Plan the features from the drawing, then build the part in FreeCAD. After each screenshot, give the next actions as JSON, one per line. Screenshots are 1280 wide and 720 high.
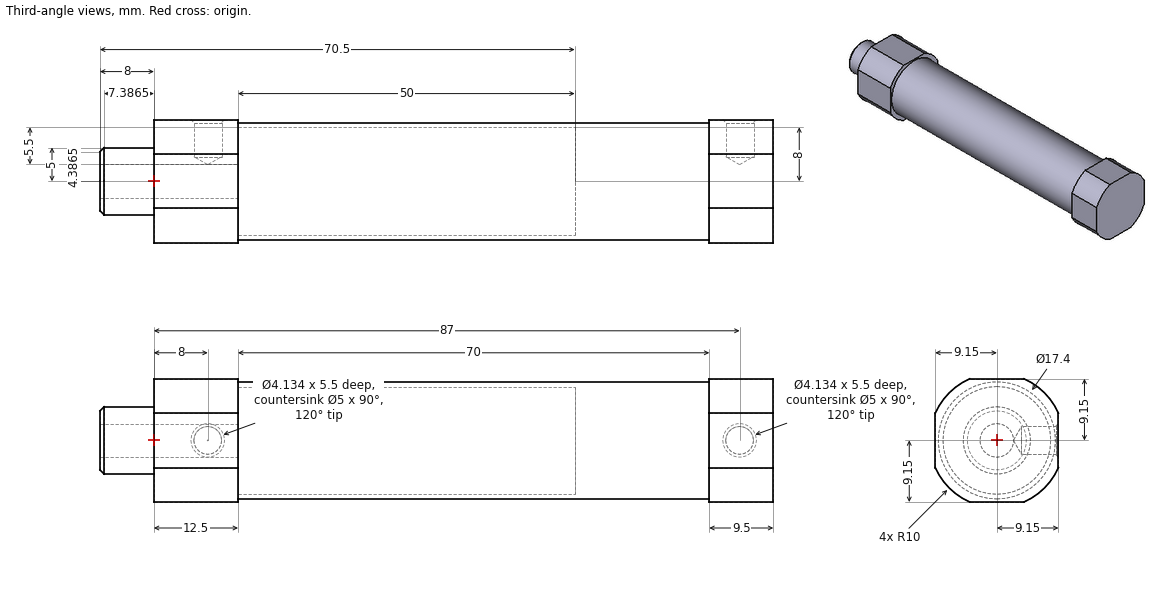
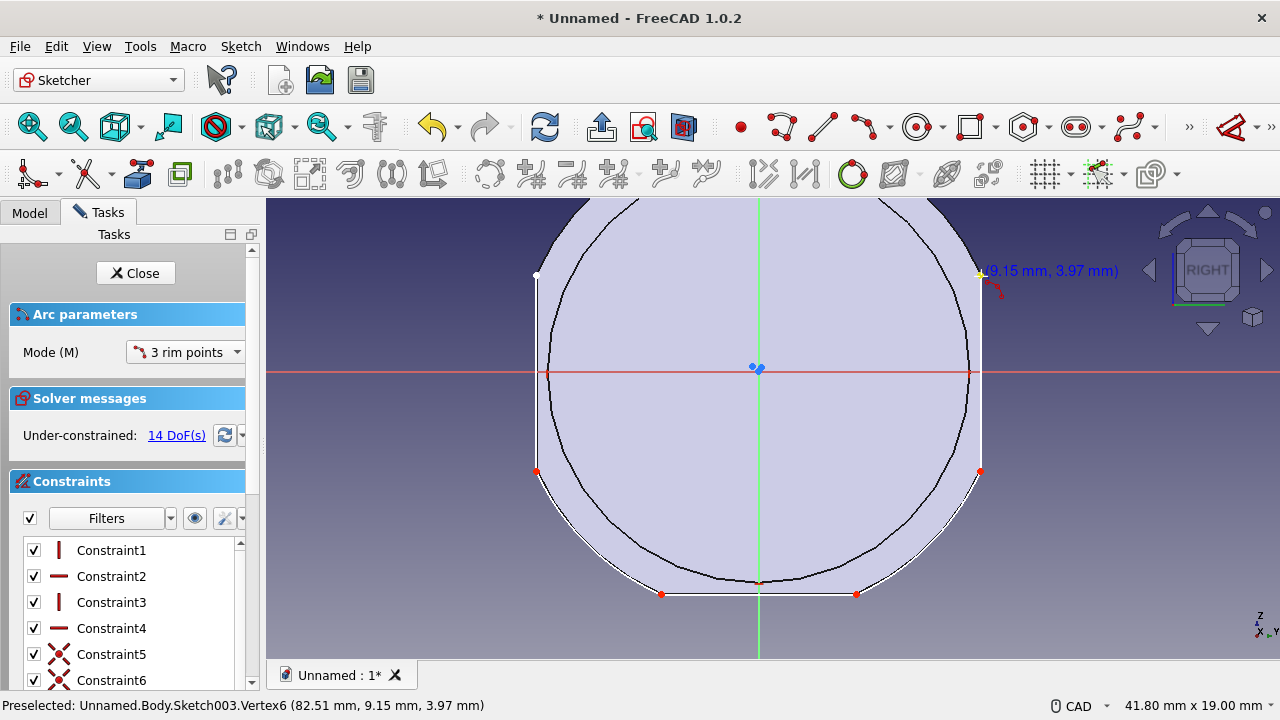
{"action": "scroll", "coordinate": [594, 544], "scroll_direction": "down", "scroll_amount": 2}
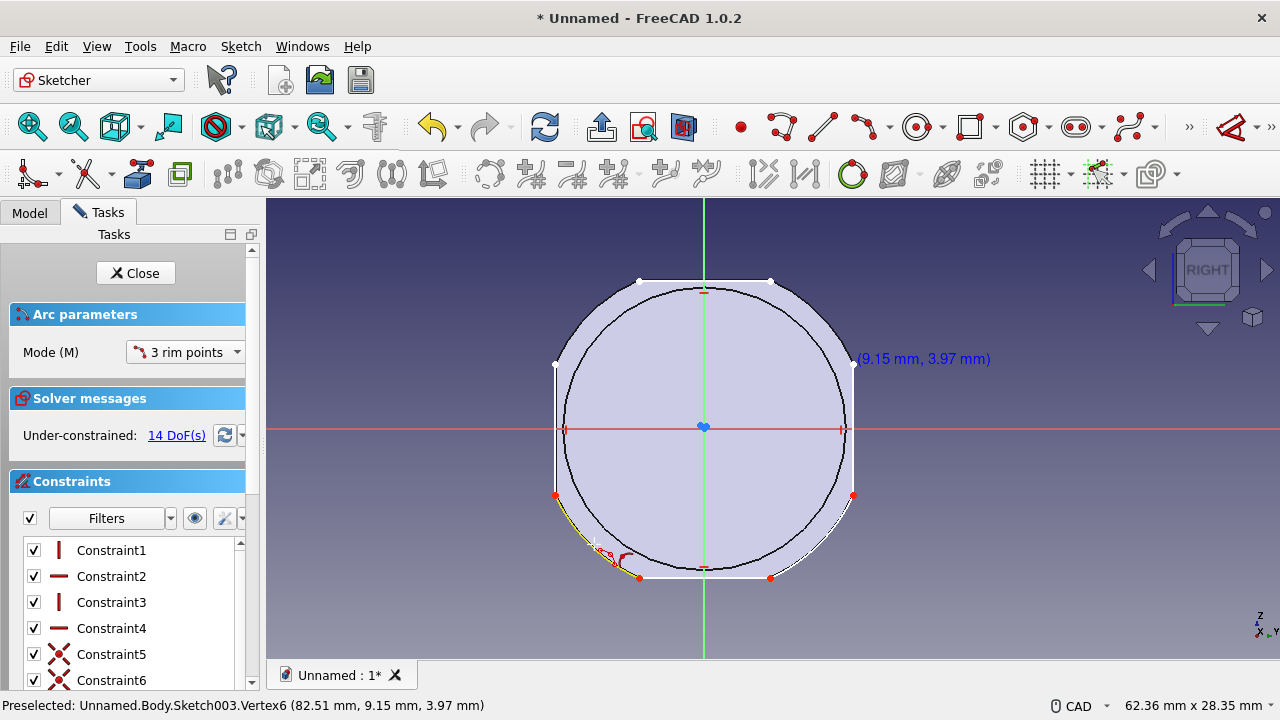
{"action": "left_click", "coordinate": [770, 281]}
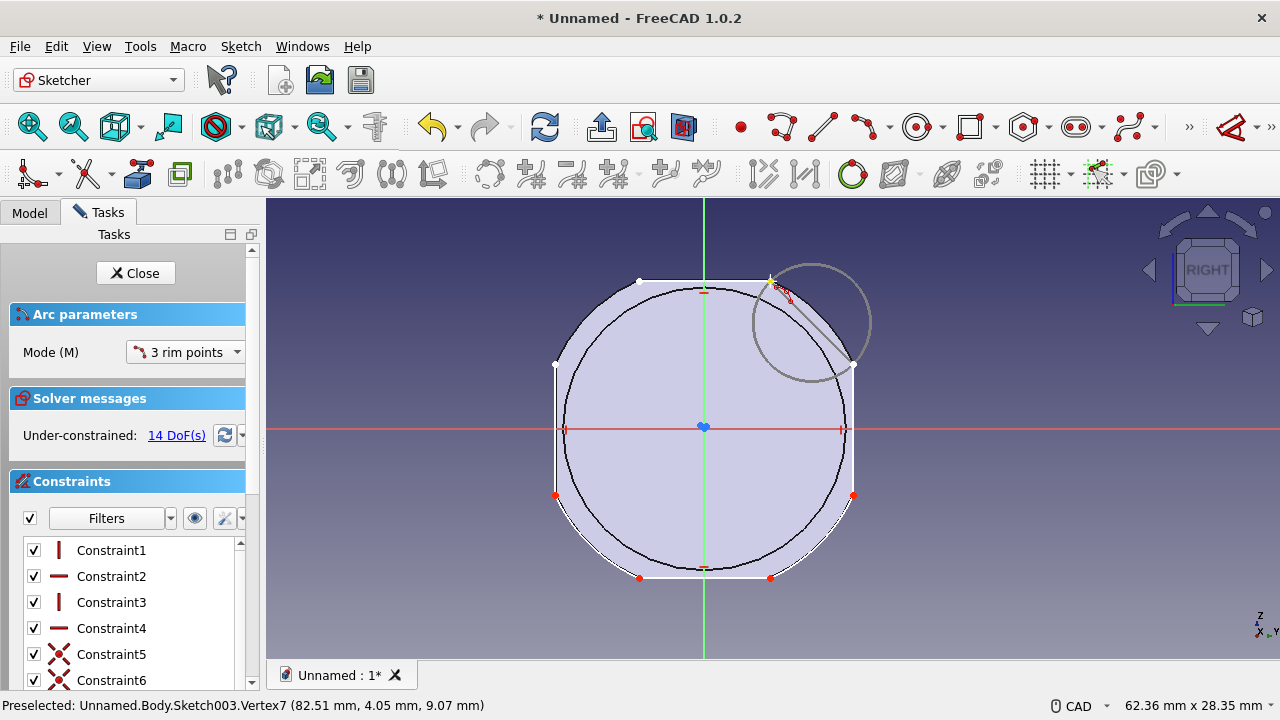
{"action": "scroll", "coordinate": [819, 314], "scroll_direction": "up", "scroll_amount": 2}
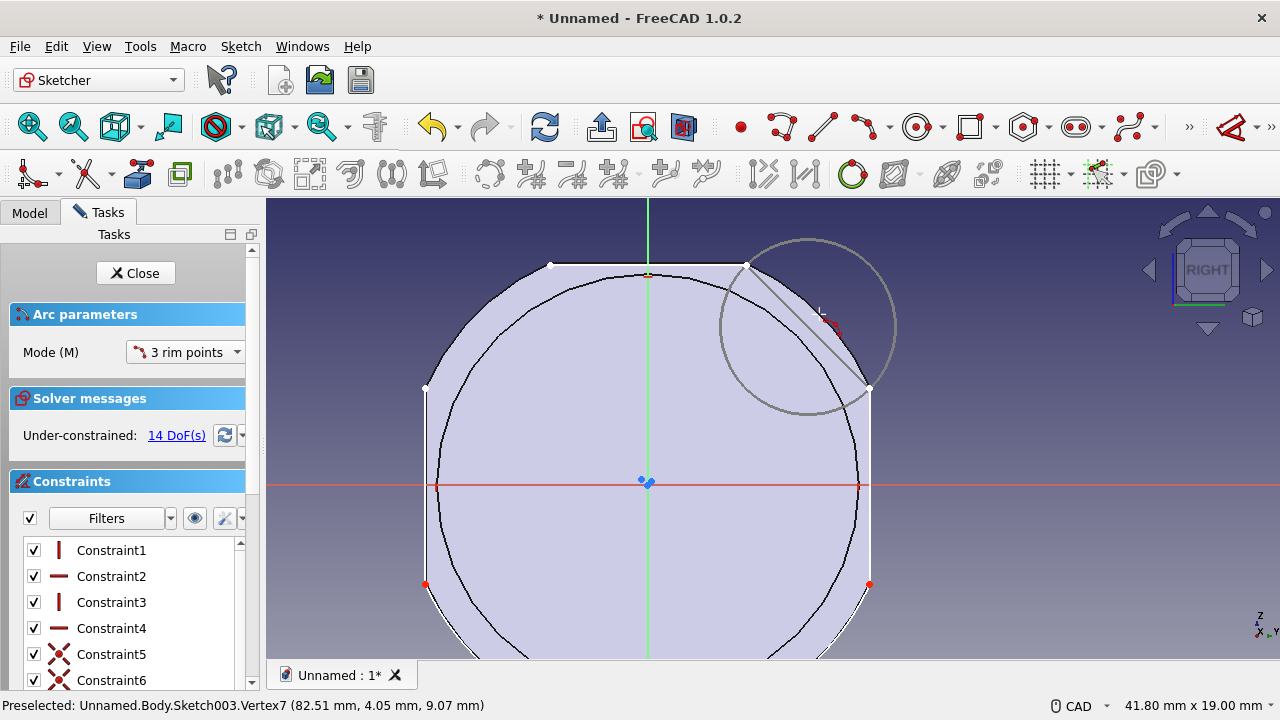
{"action": "left_click", "coordinate": [819, 314]}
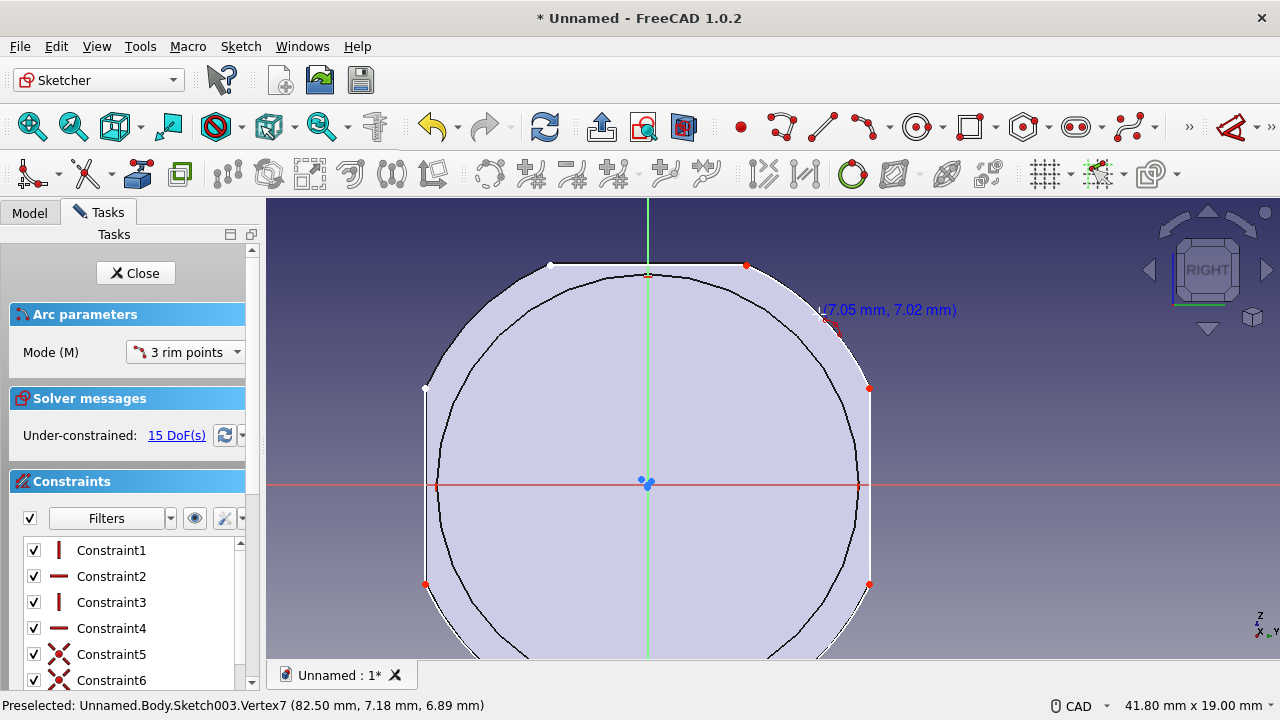
{"action": "left_click", "coordinate": [551, 265]}
{"action": "left_click", "coordinate": [425, 389]}
{"action": "left_click", "coordinate": [476, 314]}
{"action": "key", "text": "Escape"}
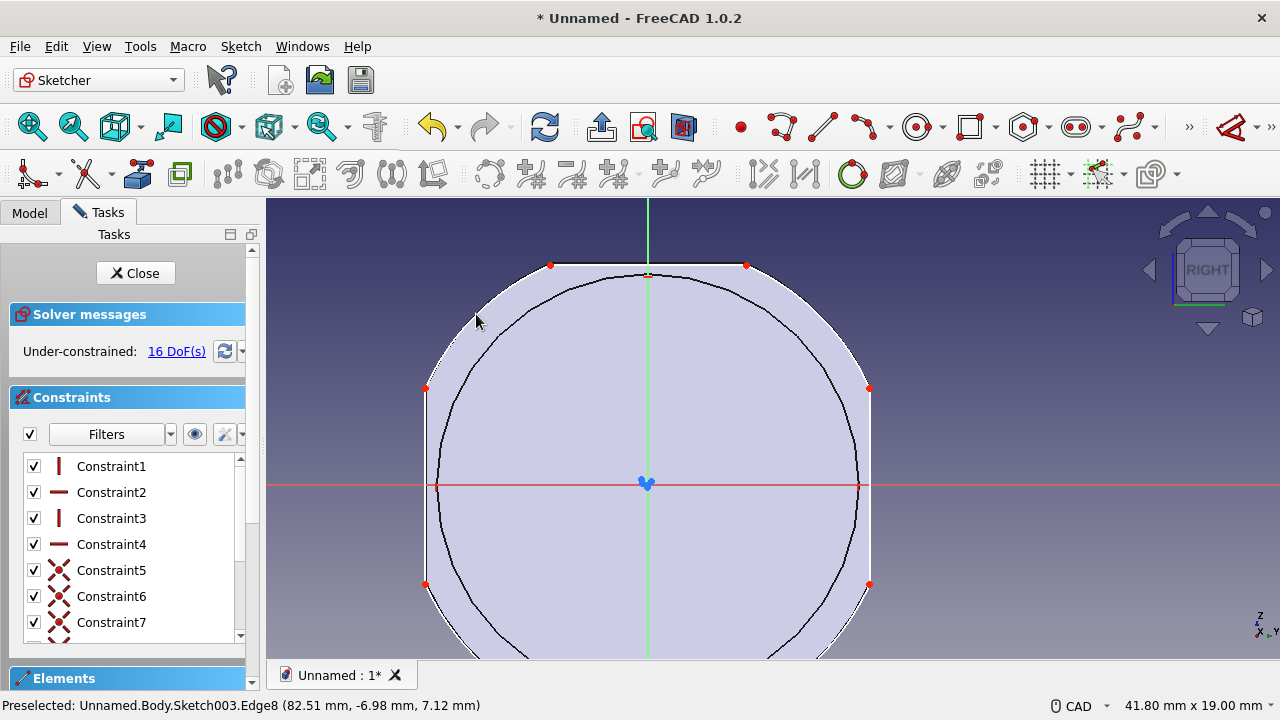
{"action": "left_click", "coordinate": [453, 631]}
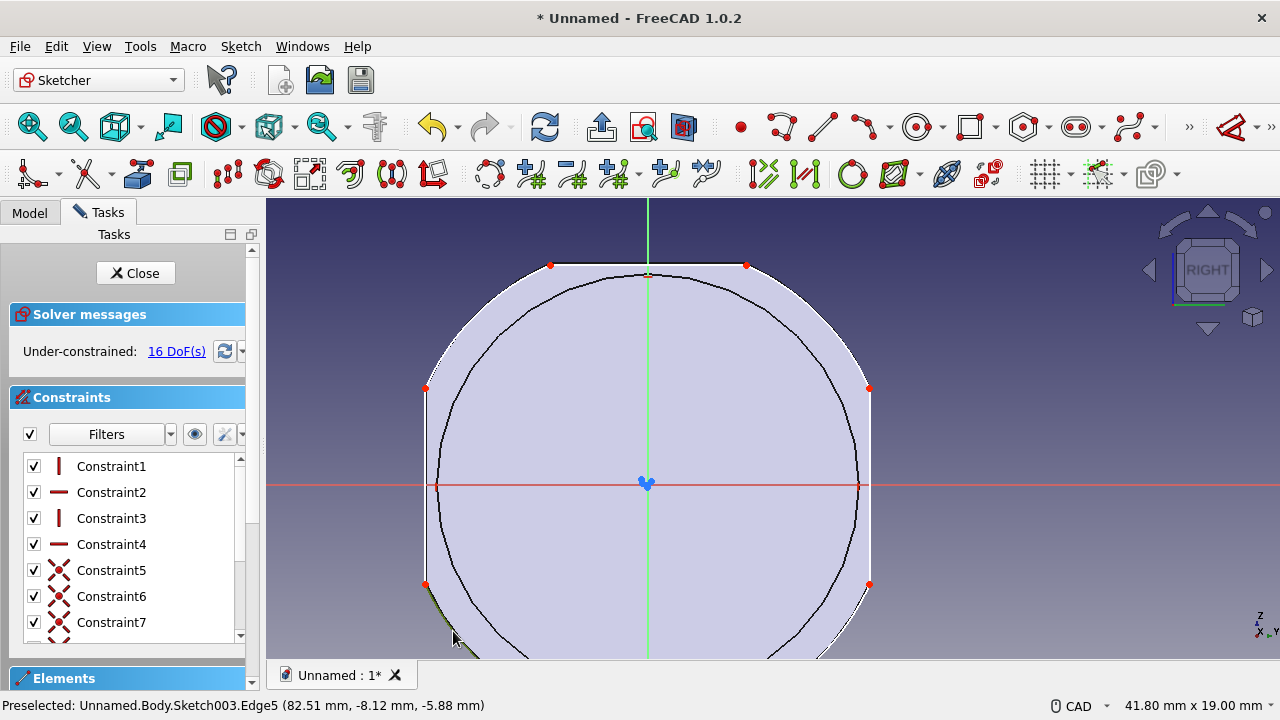
{"action": "left_click", "coordinate": [843, 630]}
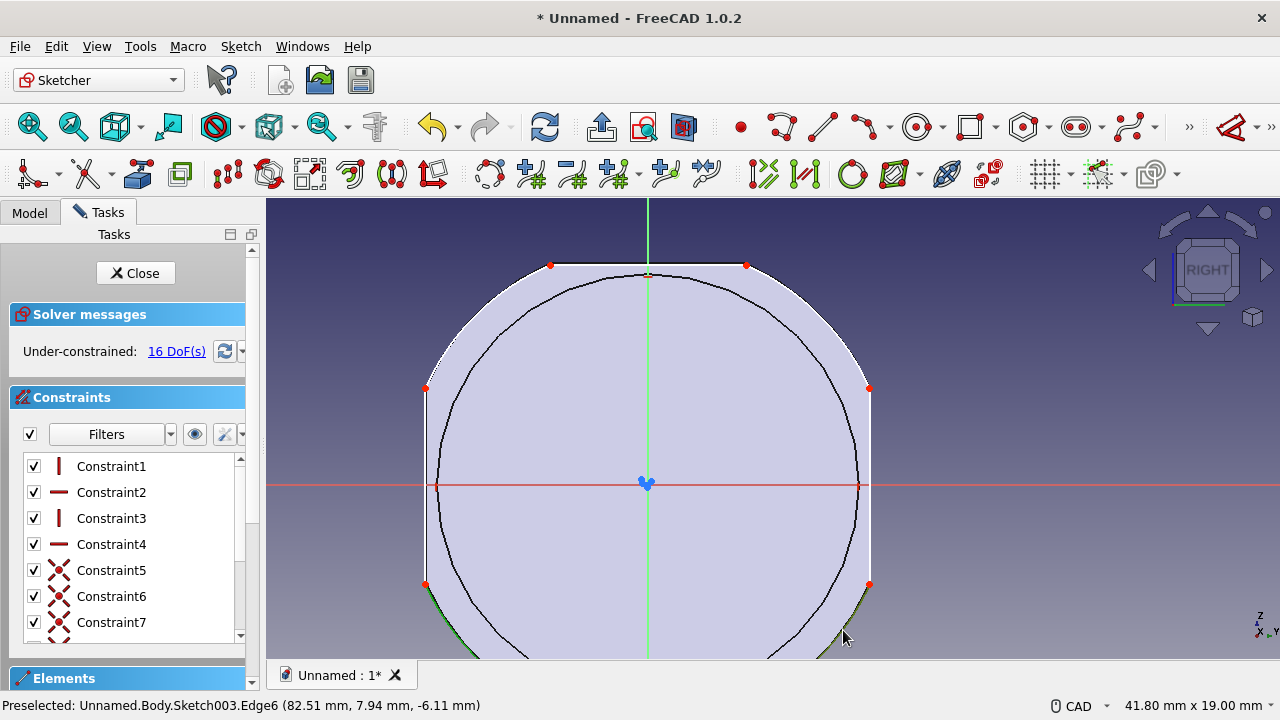
{"action": "key", "text": "c"}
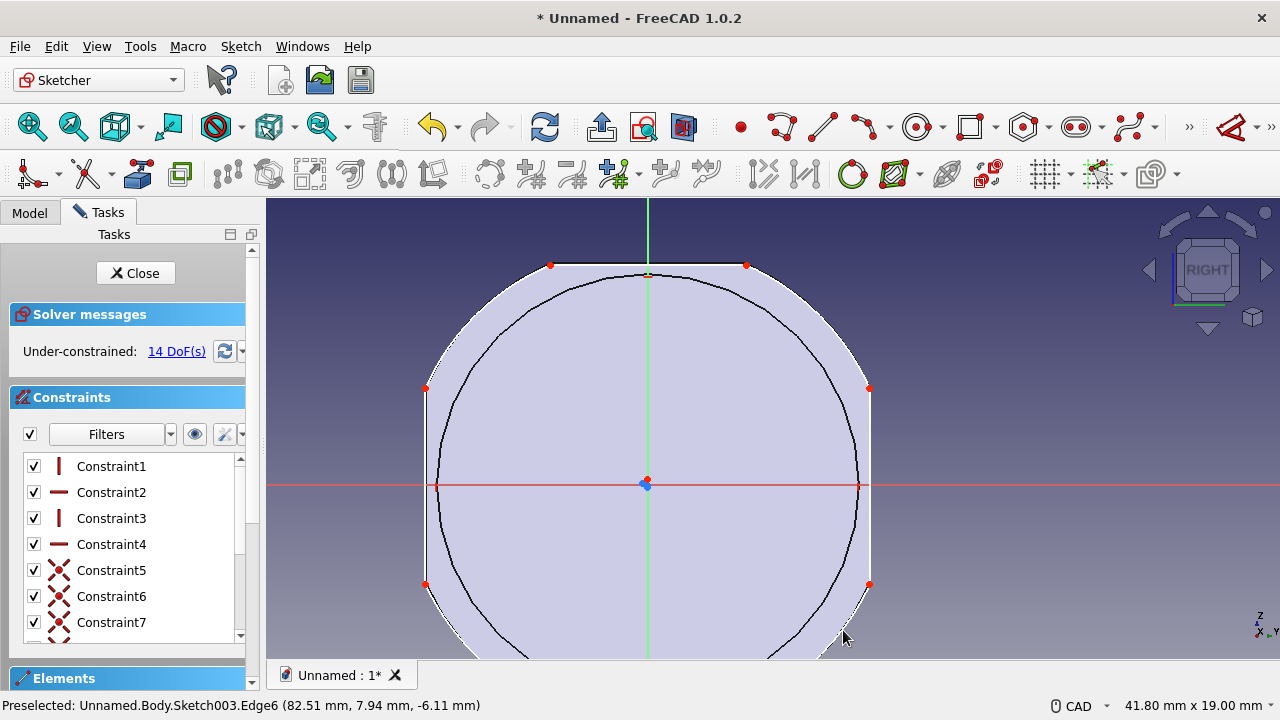
{"action": "left_click", "coordinate": [453, 630]}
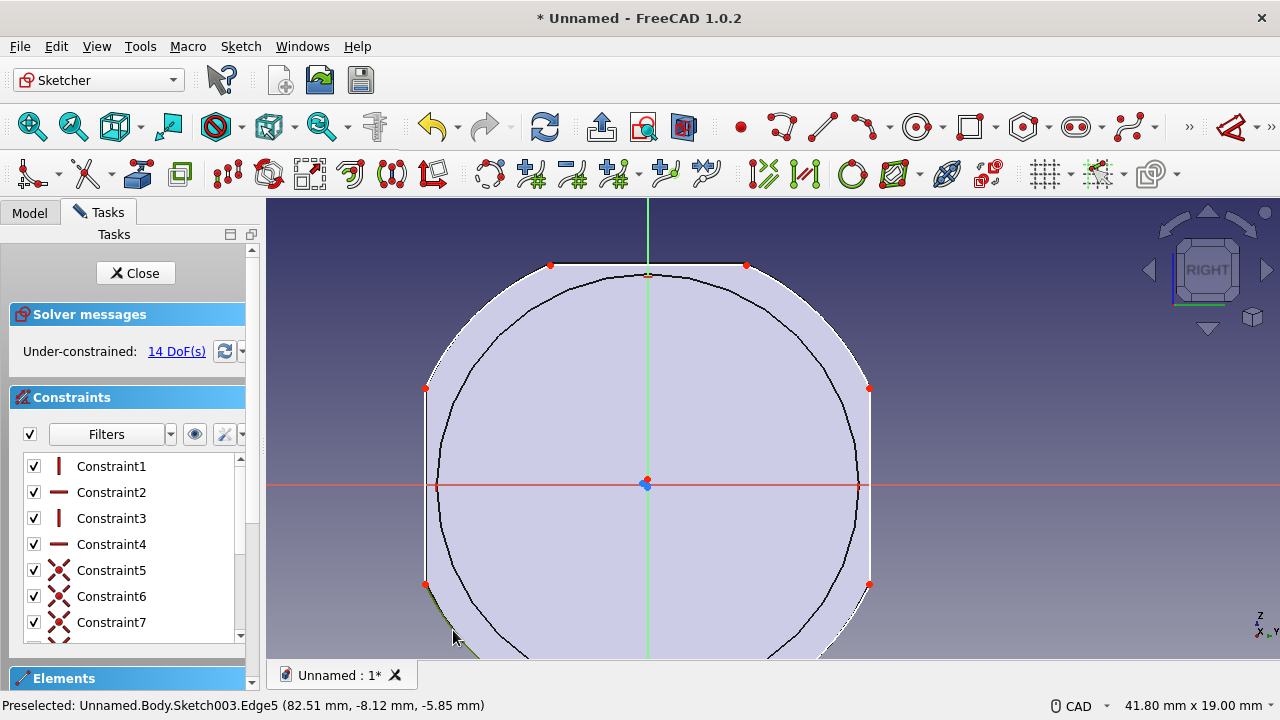
{"action": "left_click", "coordinate": [843, 343]}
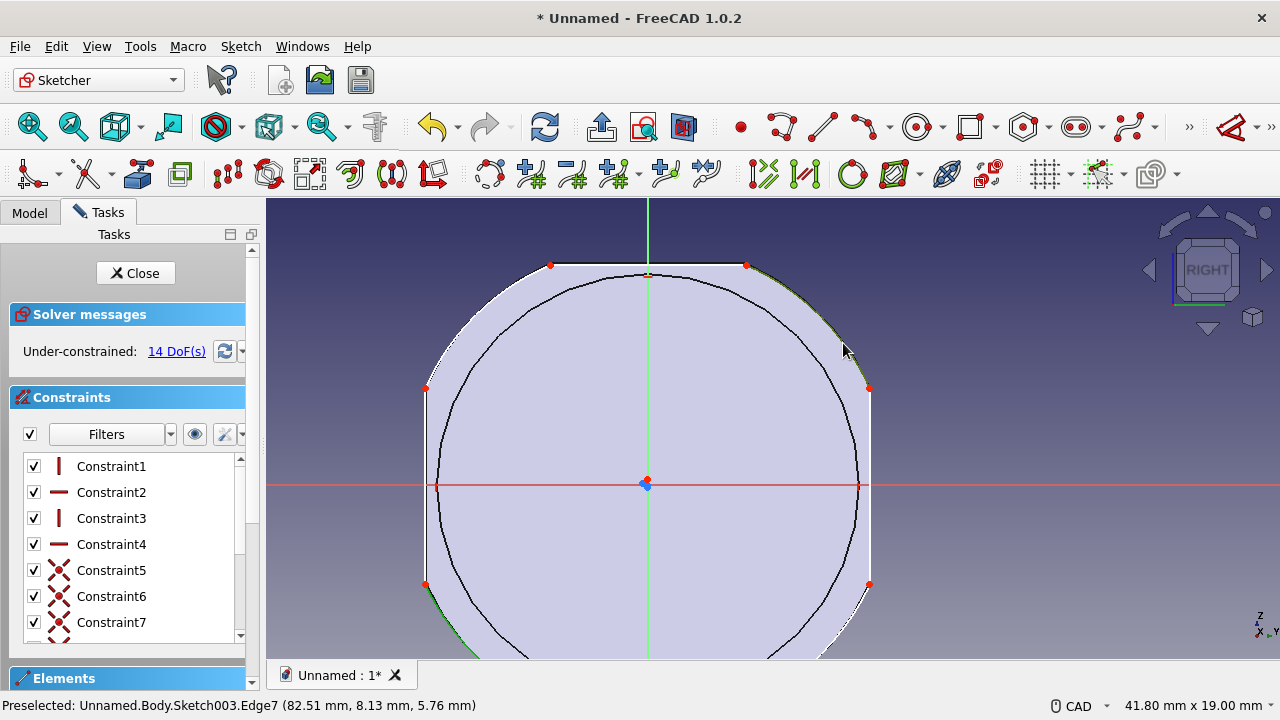
{"action": "key", "text": "c"}